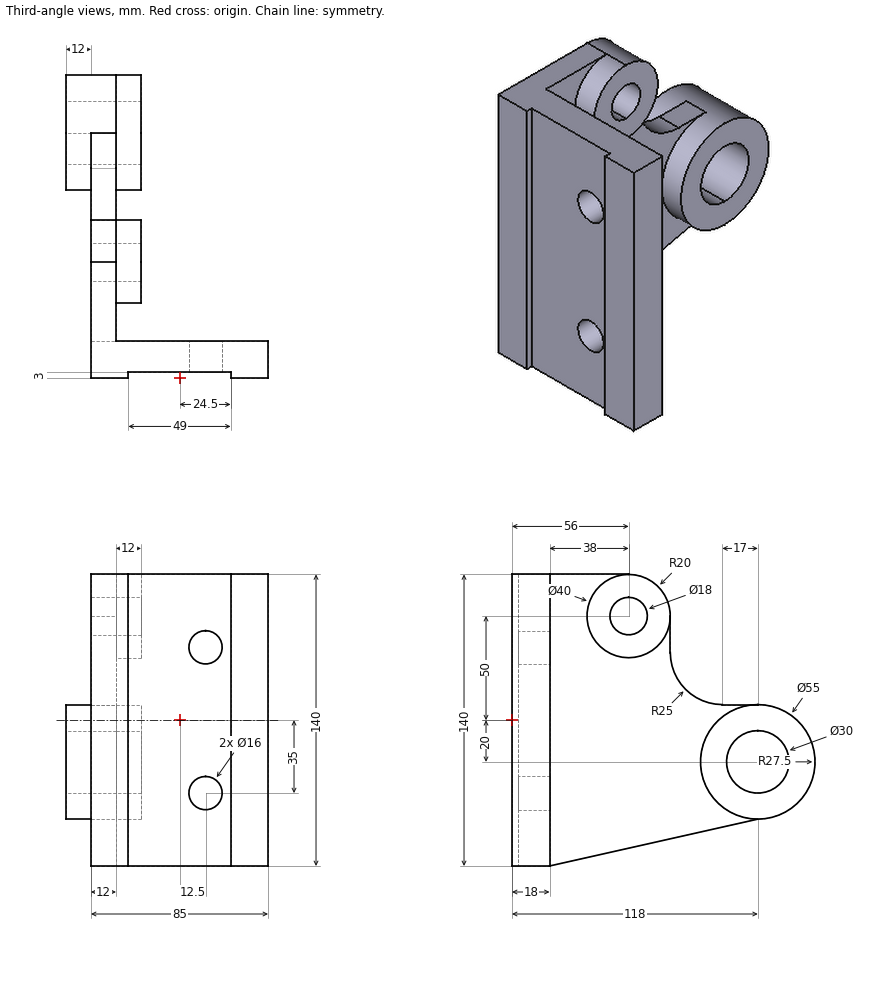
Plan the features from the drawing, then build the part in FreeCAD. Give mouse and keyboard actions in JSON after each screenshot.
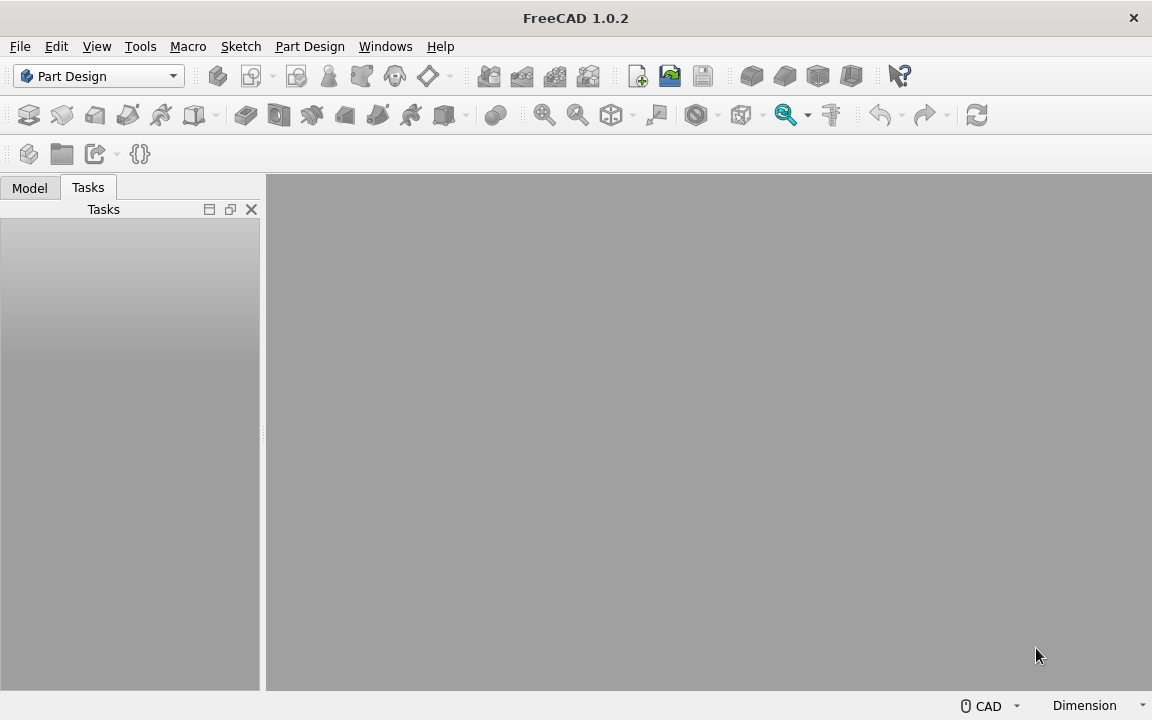
{"action": "left_click", "coordinate": [637, 76]}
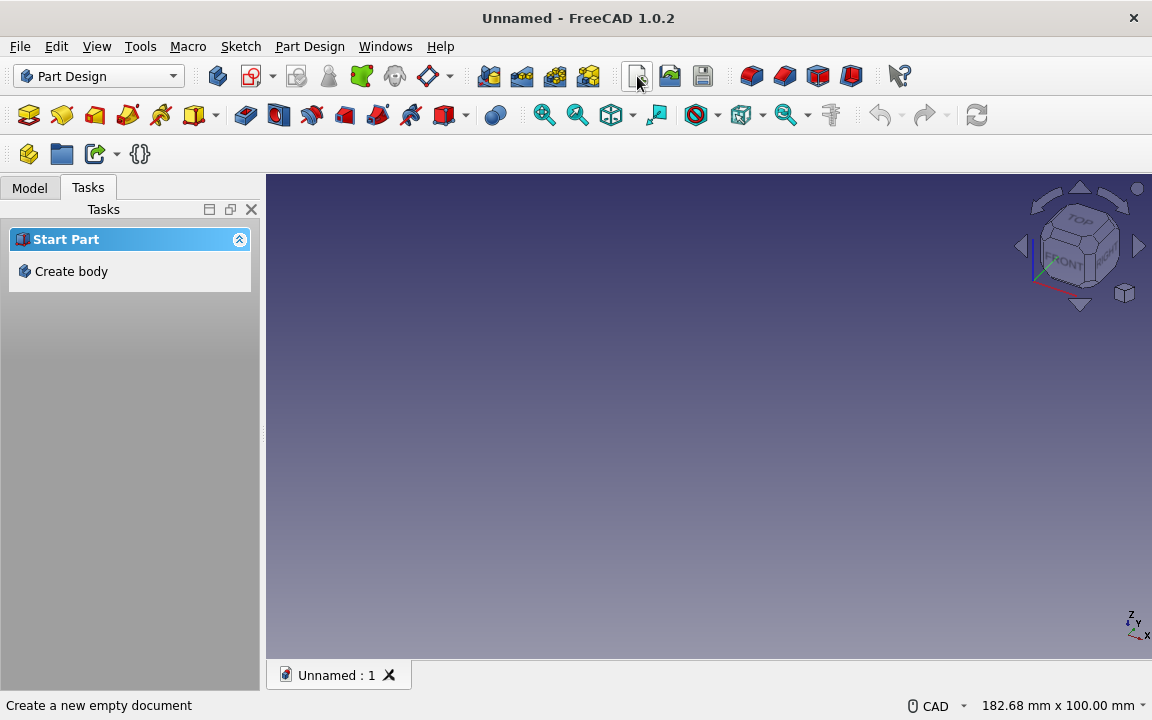
{"action": "left_click", "coordinate": [250, 76]}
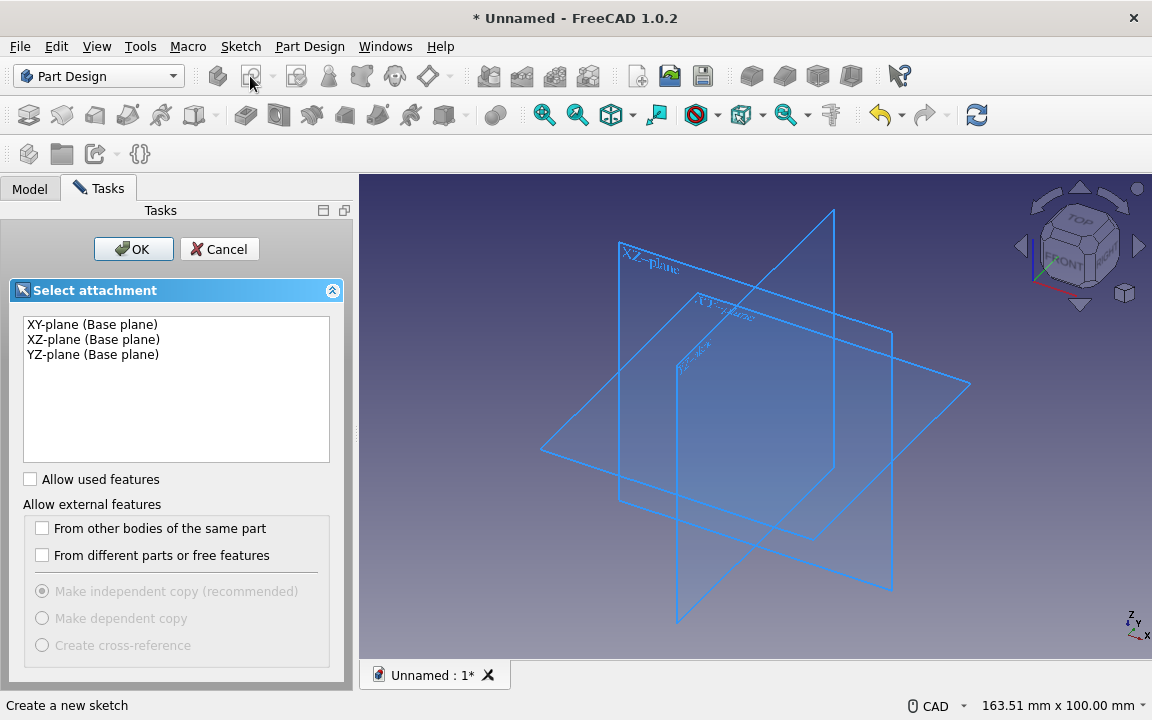
{"action": "left_click", "coordinate": [84, 340]}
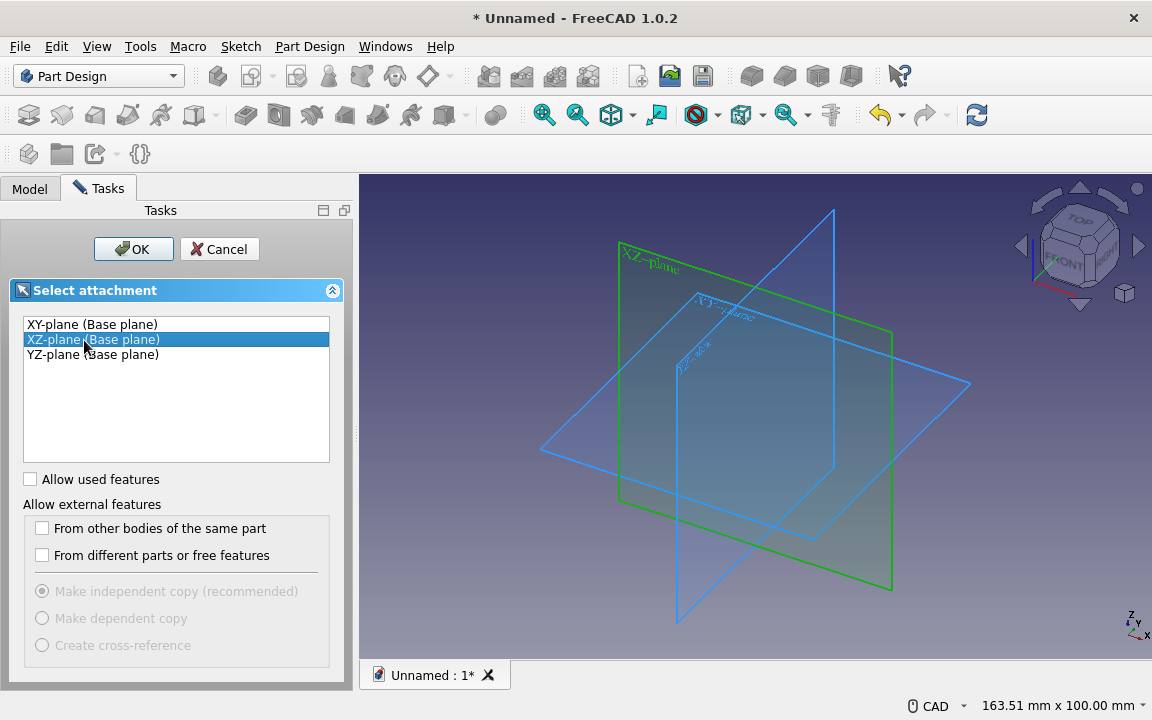
{"action": "left_click", "coordinate": [134, 249]}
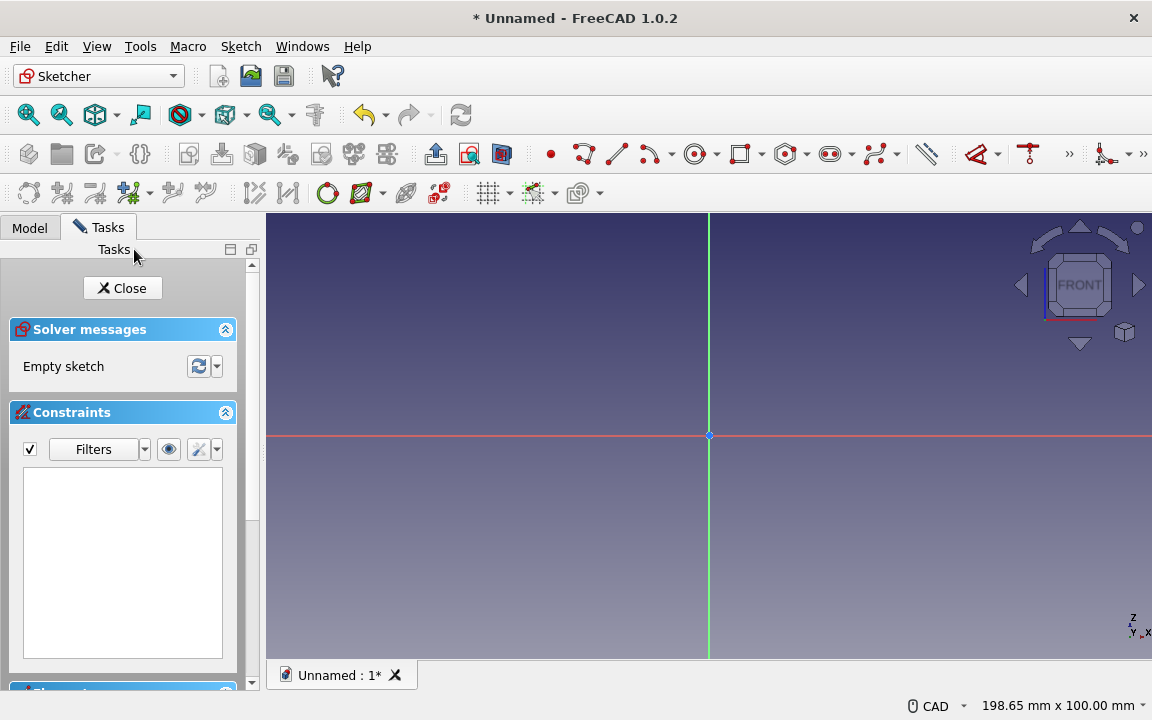
{"action": "scroll", "coordinate": [585, 436], "scroll_direction": "down", "scroll_amount": 4}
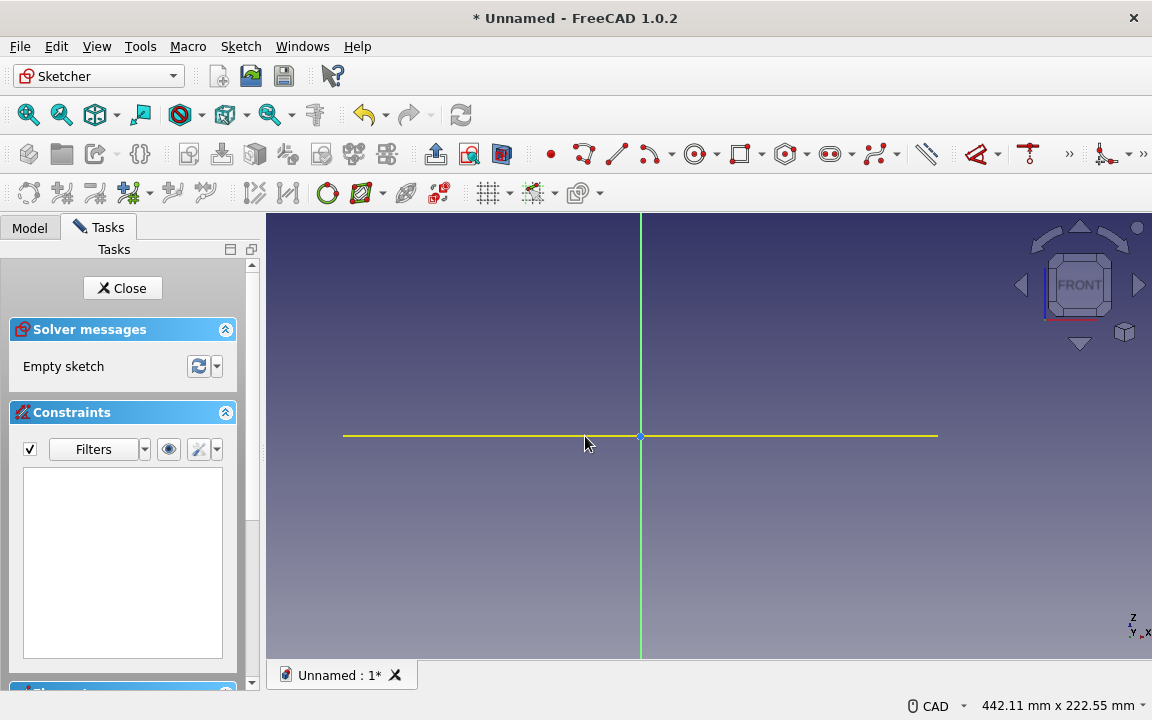
{"action": "key", "text": "g v"}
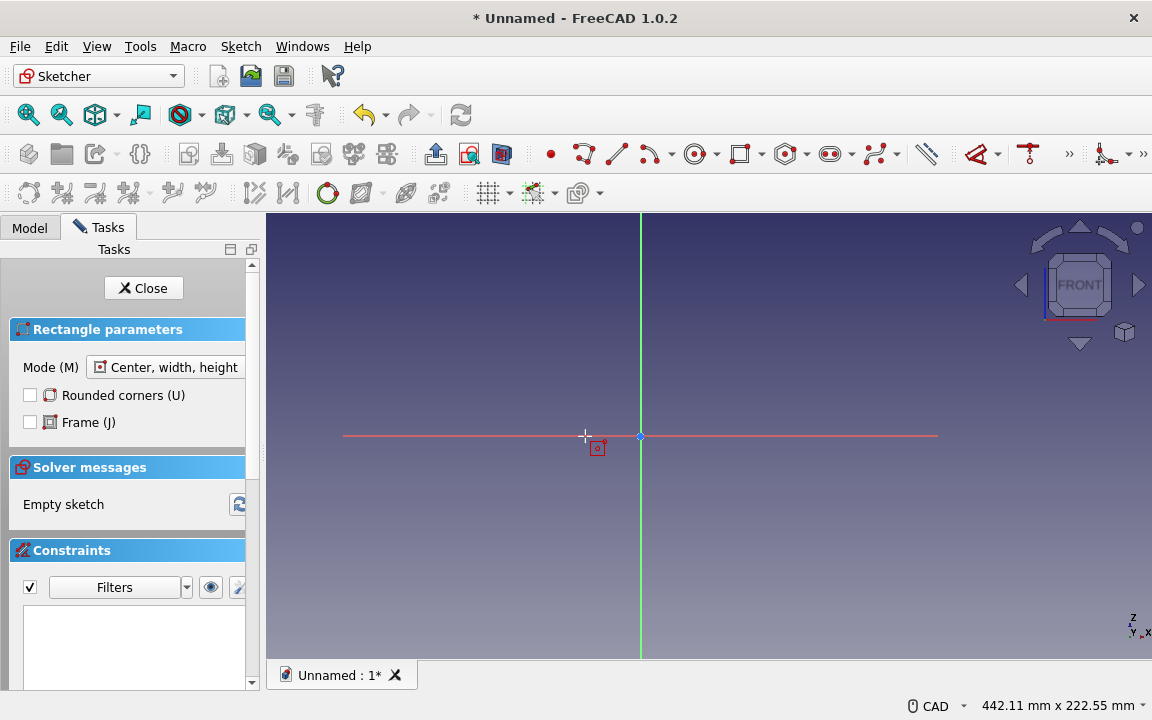
{"action": "left_click", "coordinate": [641, 436]}
{"action": "mouse_move", "coordinate": [726, 296]}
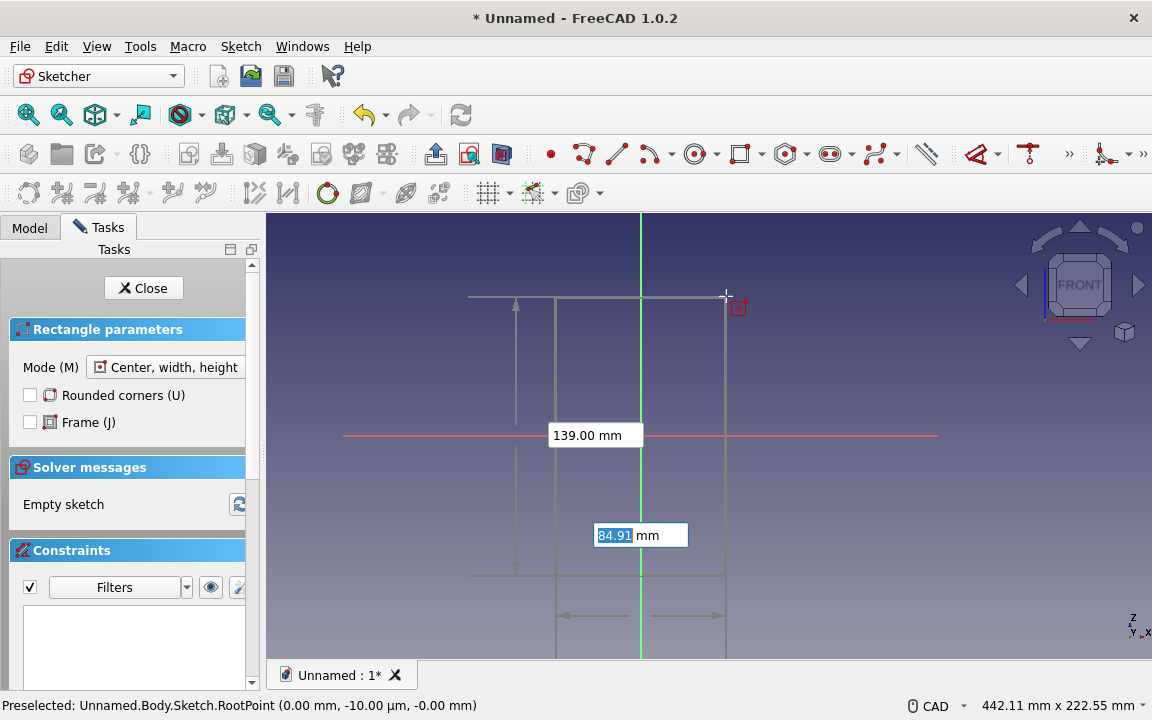
{"action": "type", "text": "85"}
{"action": "key", "text": "Tab"}
{"action": "type", "text": "140"}
{"action": "key", "text": "Return"}
{"action": "key", "text": "Escape"}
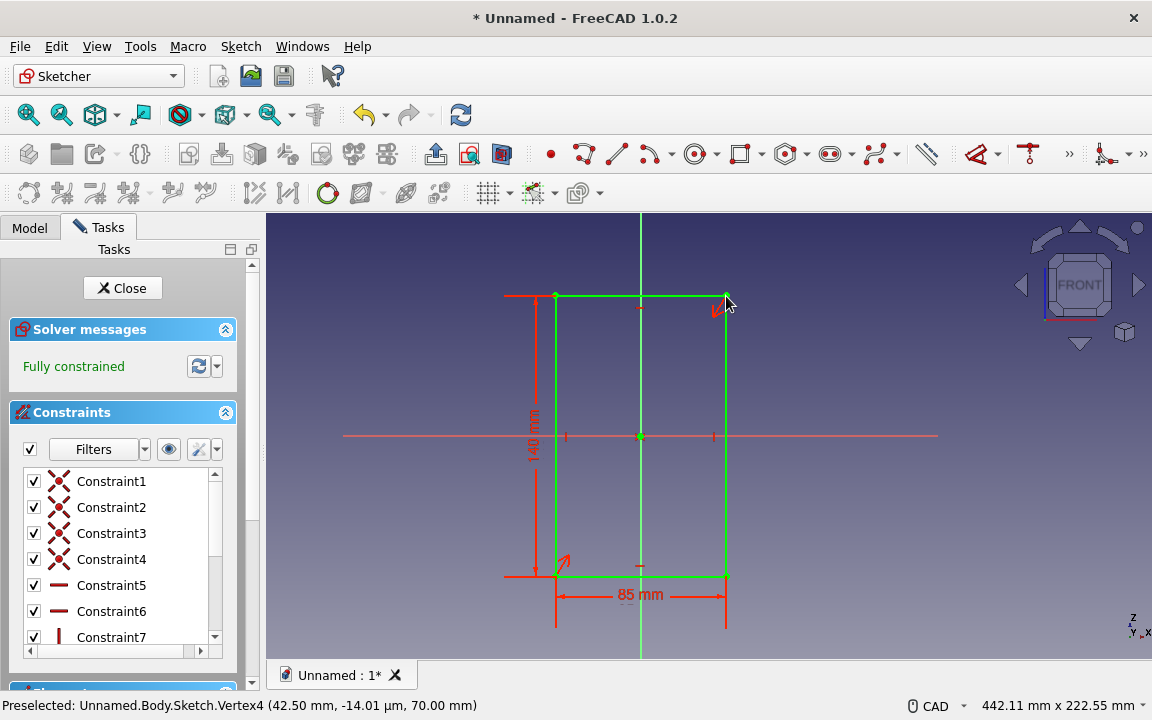
{"action": "left_click", "coordinate": [123, 288]}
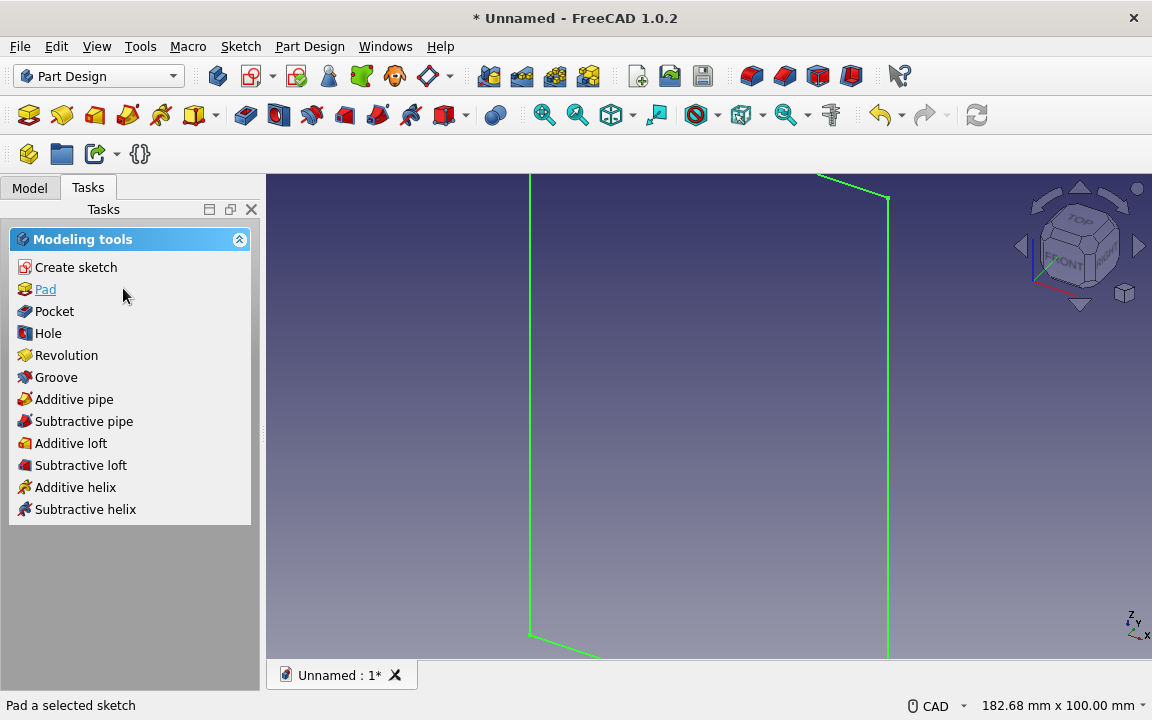
{"action": "left_click", "coordinate": [29, 116]}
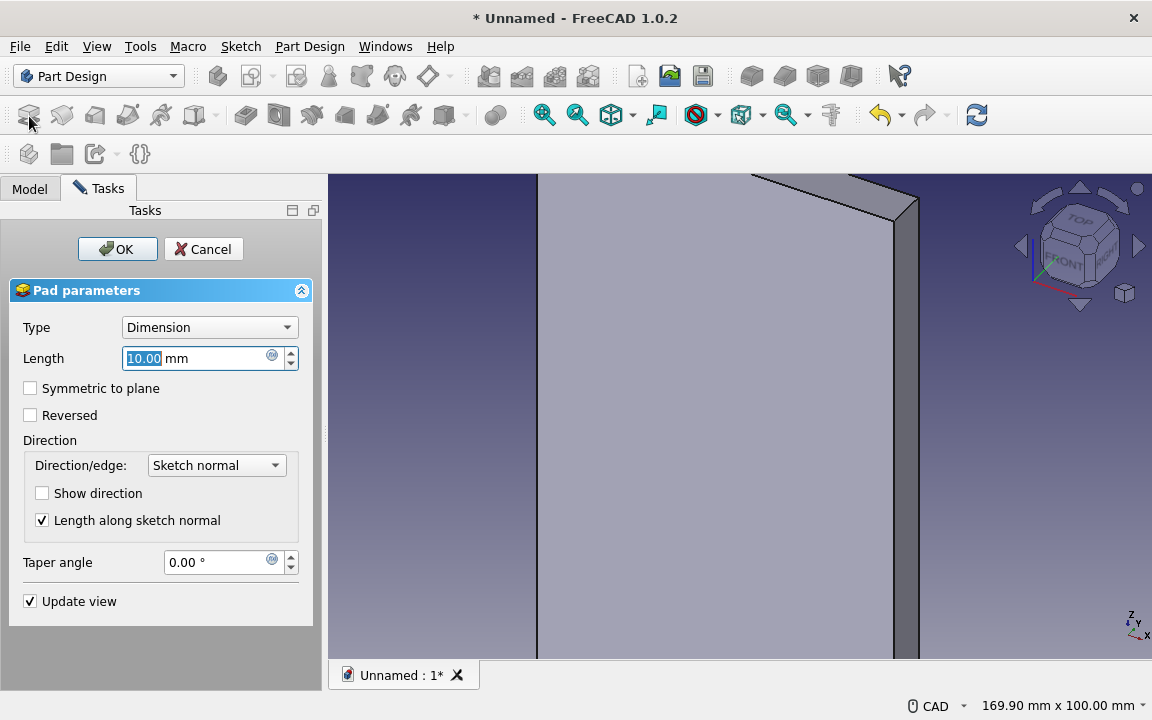
{"action": "type", "text": "18"}
{"action": "key", "text": "Tab"}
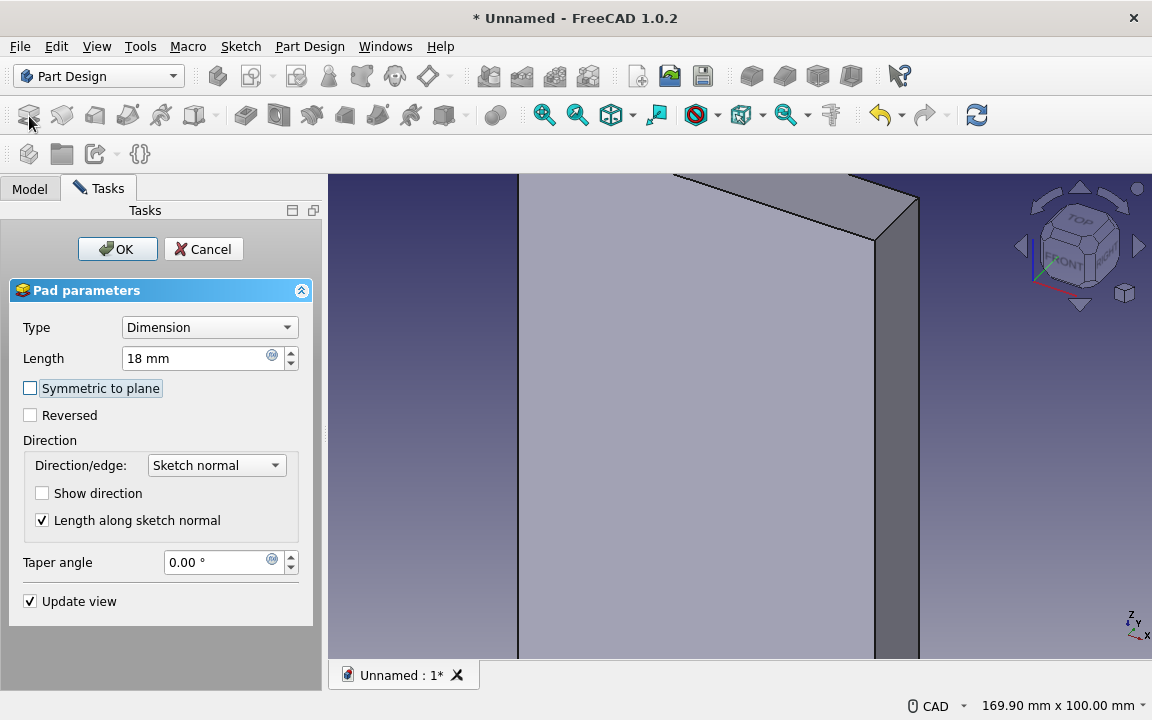
{"action": "left_click", "coordinate": [31, 415]}